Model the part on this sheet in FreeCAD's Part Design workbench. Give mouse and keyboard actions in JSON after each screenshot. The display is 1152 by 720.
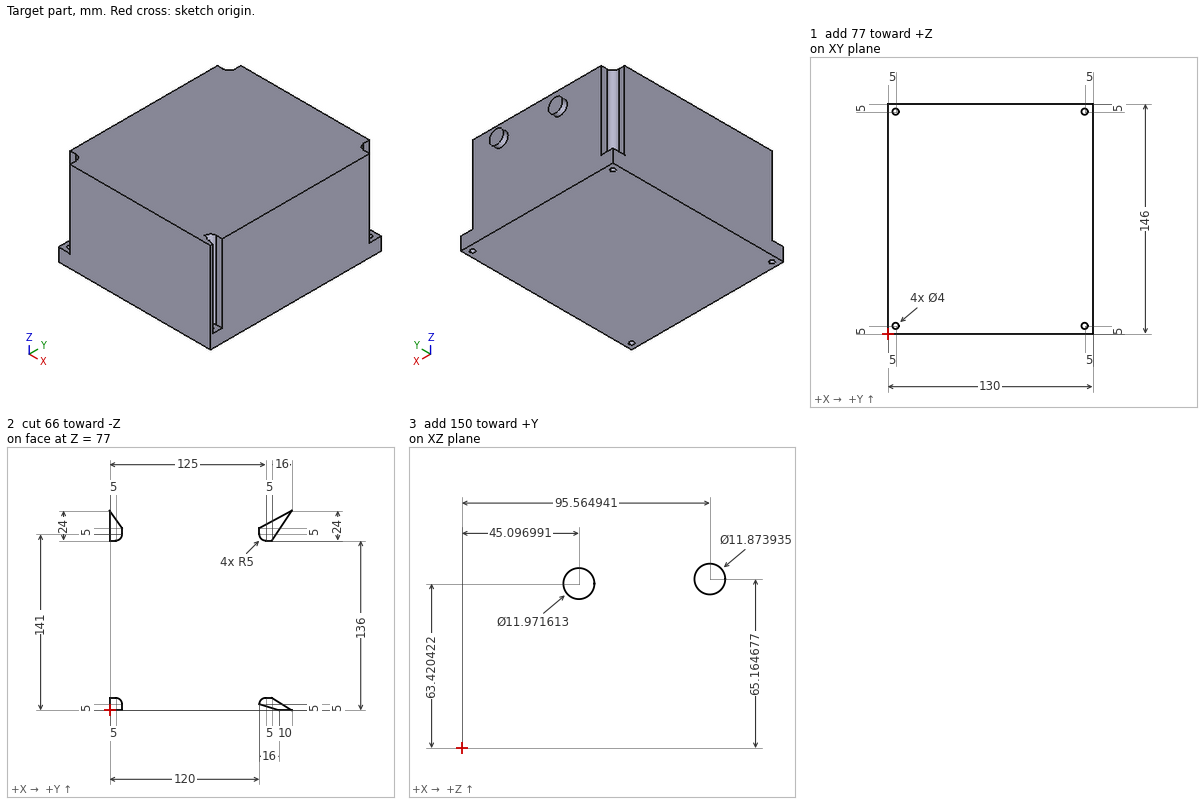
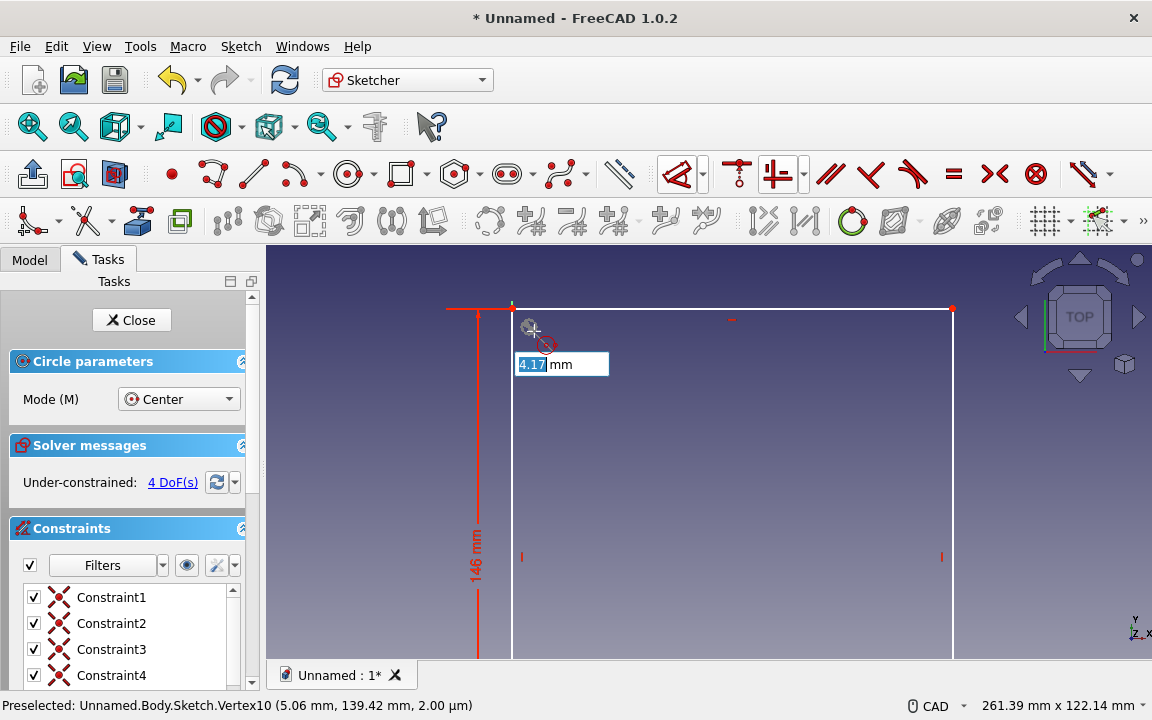
{"action": "type", "text": "4"}
{"action": "key", "text": "Return"}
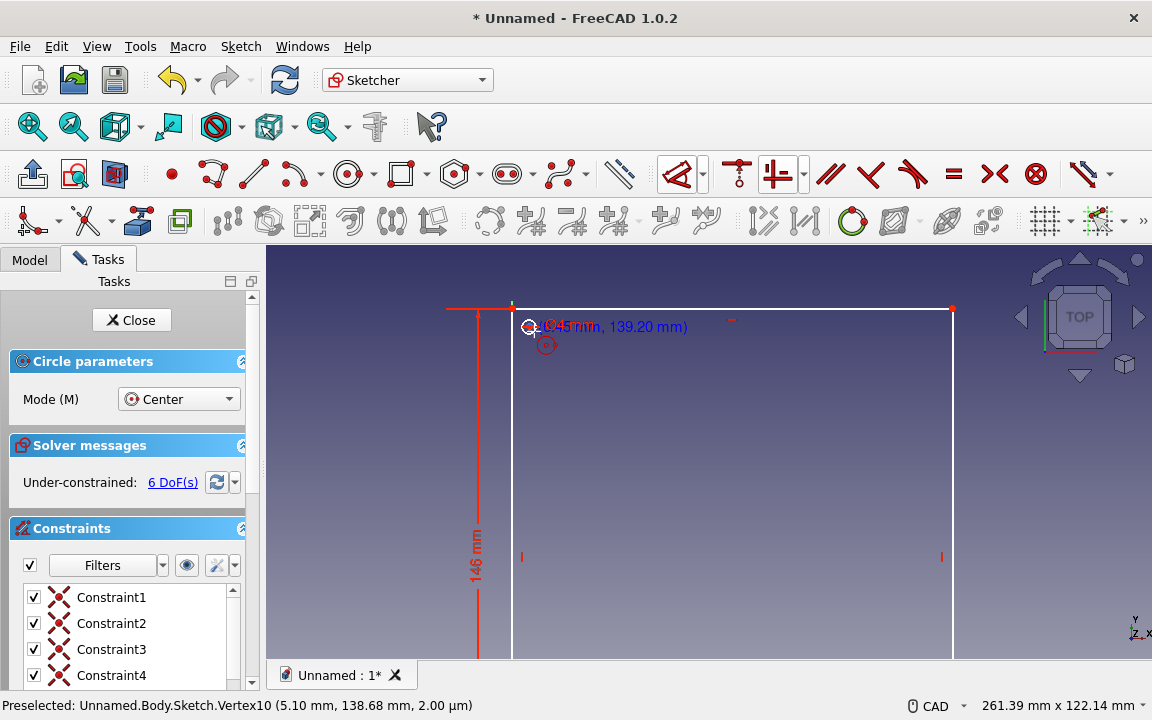
{"action": "scroll", "coordinate": [936, 326], "scroll_direction": "up", "scroll_amount": 7}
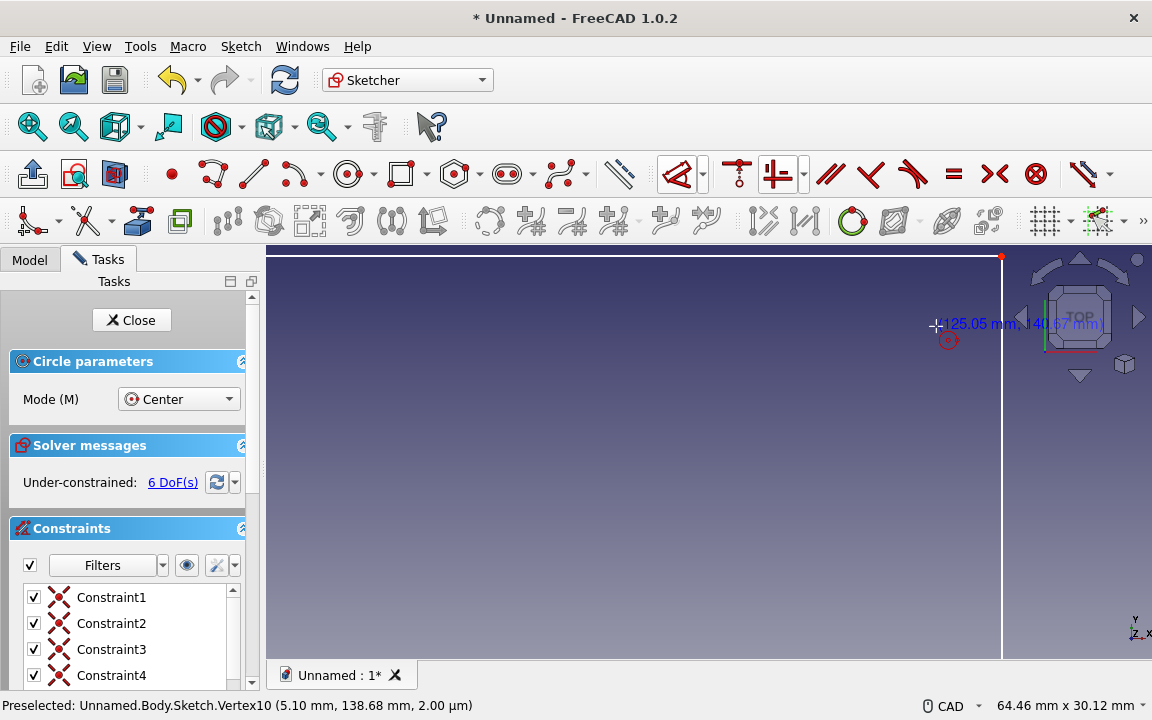
{"action": "scroll", "coordinate": [724, 326], "scroll_direction": "down", "scroll_amount": 10}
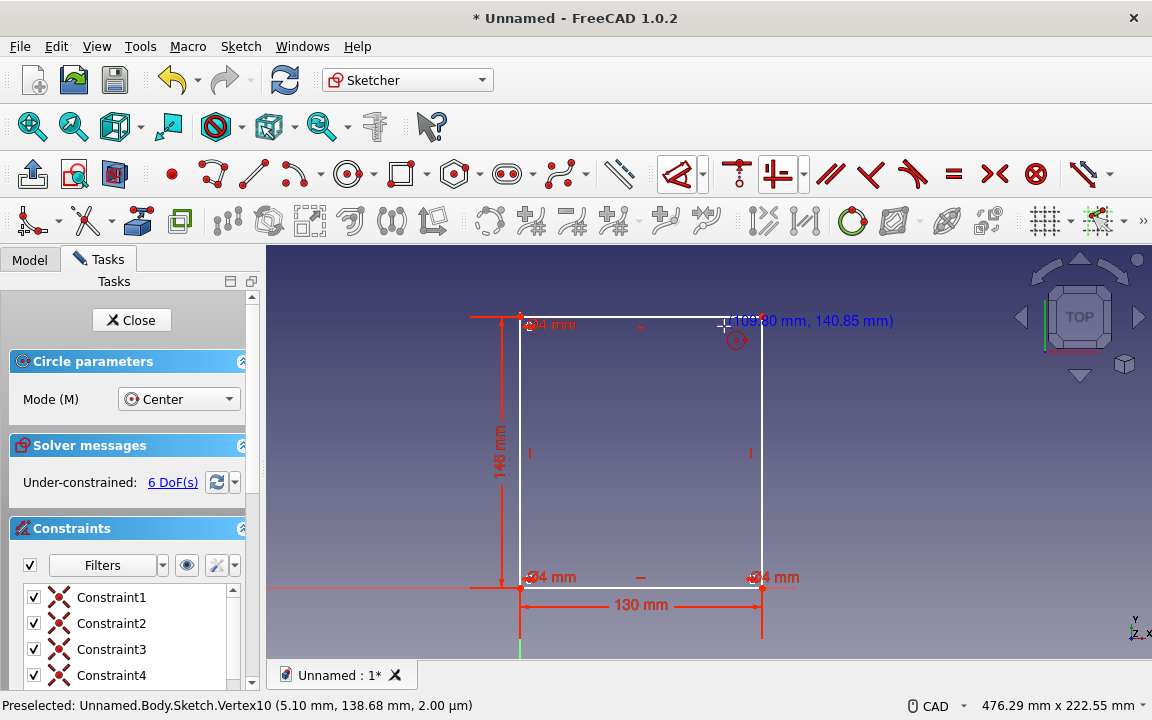
{"action": "scroll", "coordinate": [753, 326], "scroll_direction": "up", "scroll_amount": 3}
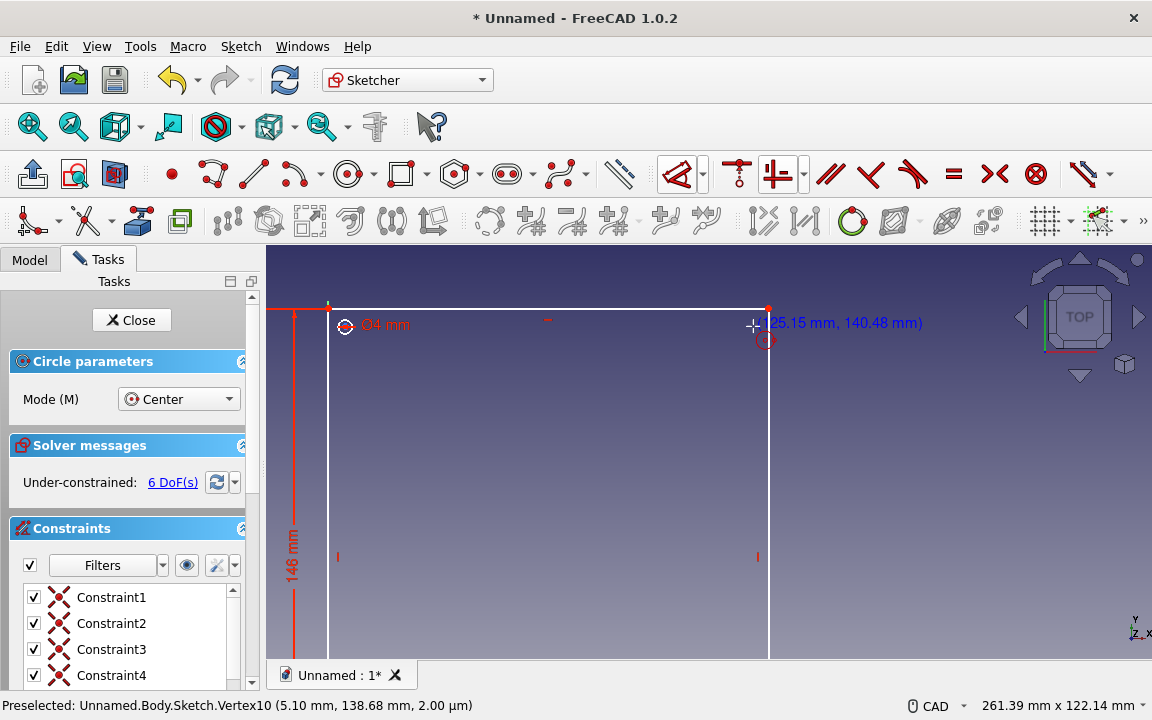
{"action": "left_click", "coordinate": [752, 326]}
{"action": "mouse_move", "coordinate": [747, 331]}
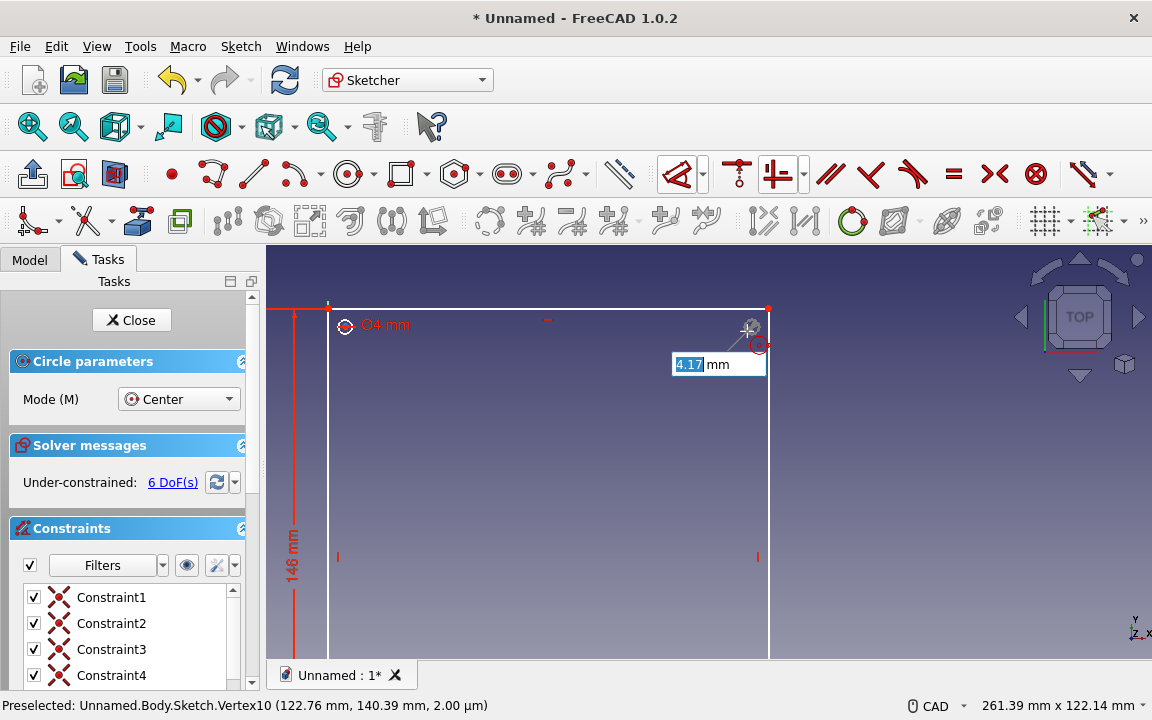
{"action": "type", "text": "4"}
{"action": "key", "text": "Return"}
{"action": "key", "text": "Escape"}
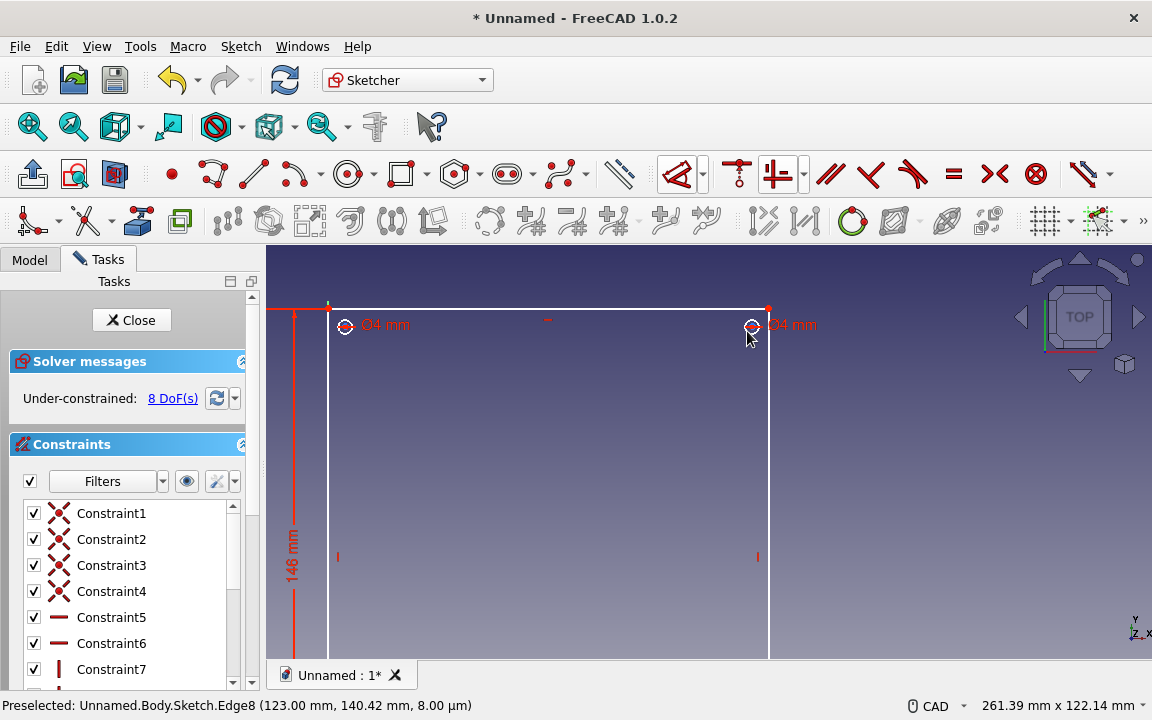
{"action": "left_click", "coordinate": [676, 174]}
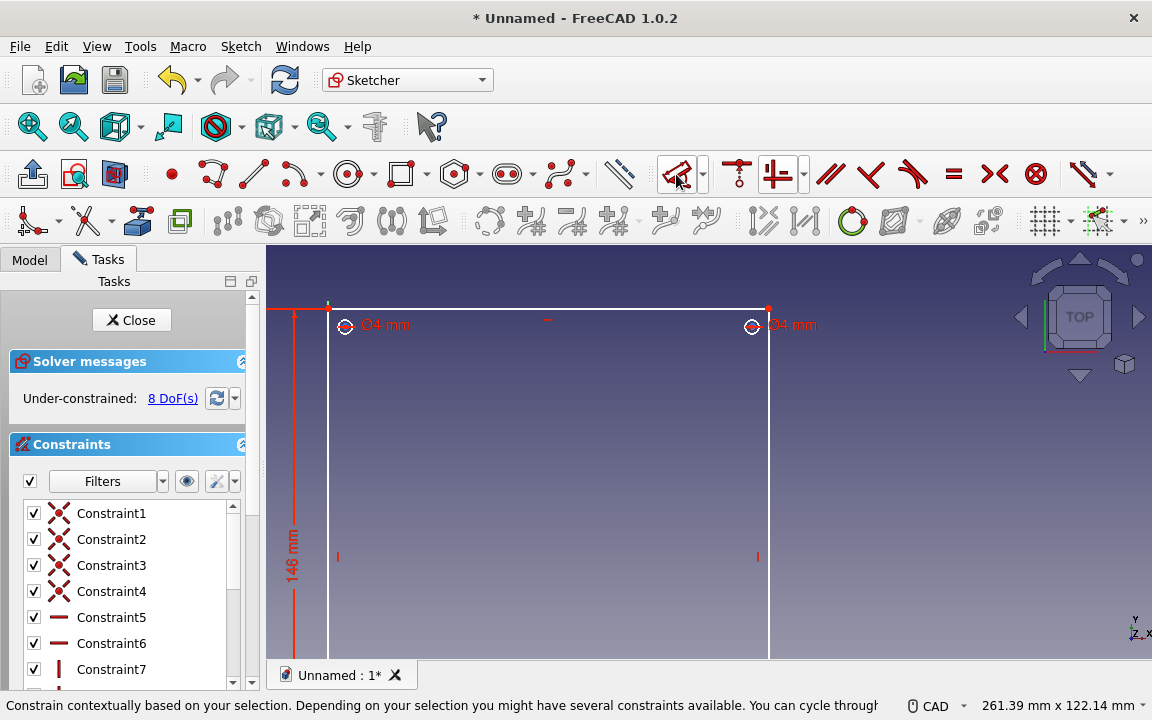
{"action": "scroll", "coordinate": [752, 325], "scroll_direction": "down", "scroll_amount": 3}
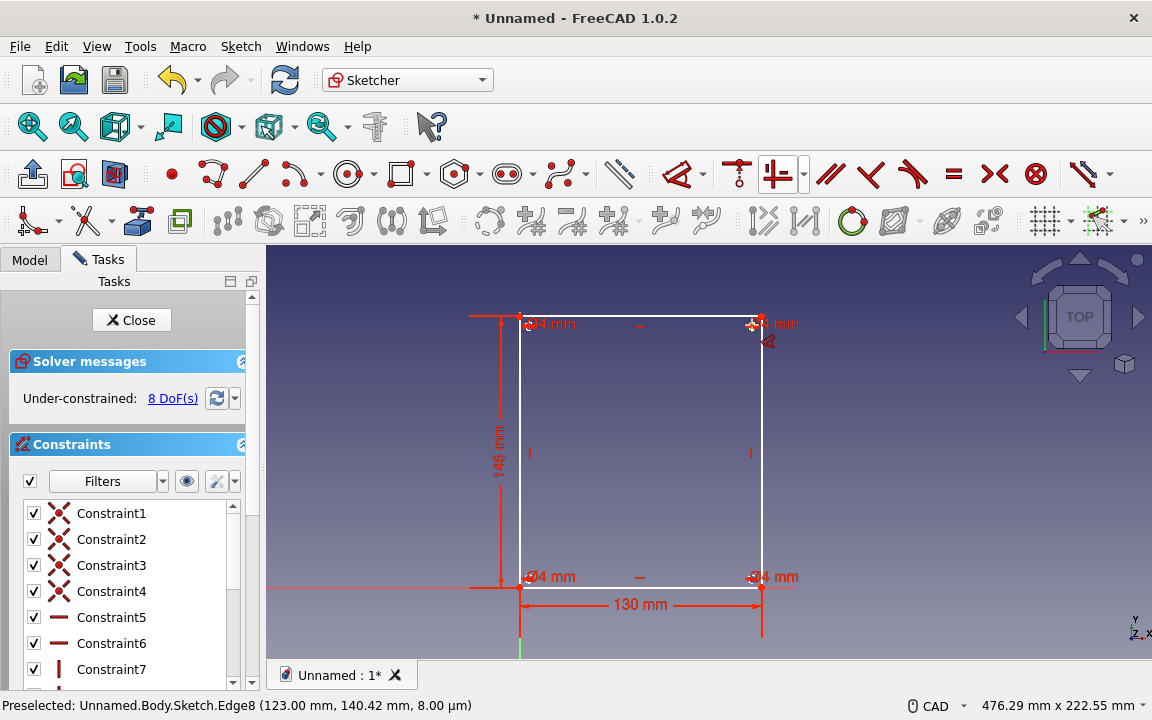
{"action": "scroll", "coordinate": [529, 579], "scroll_direction": "up", "scroll_amount": 8}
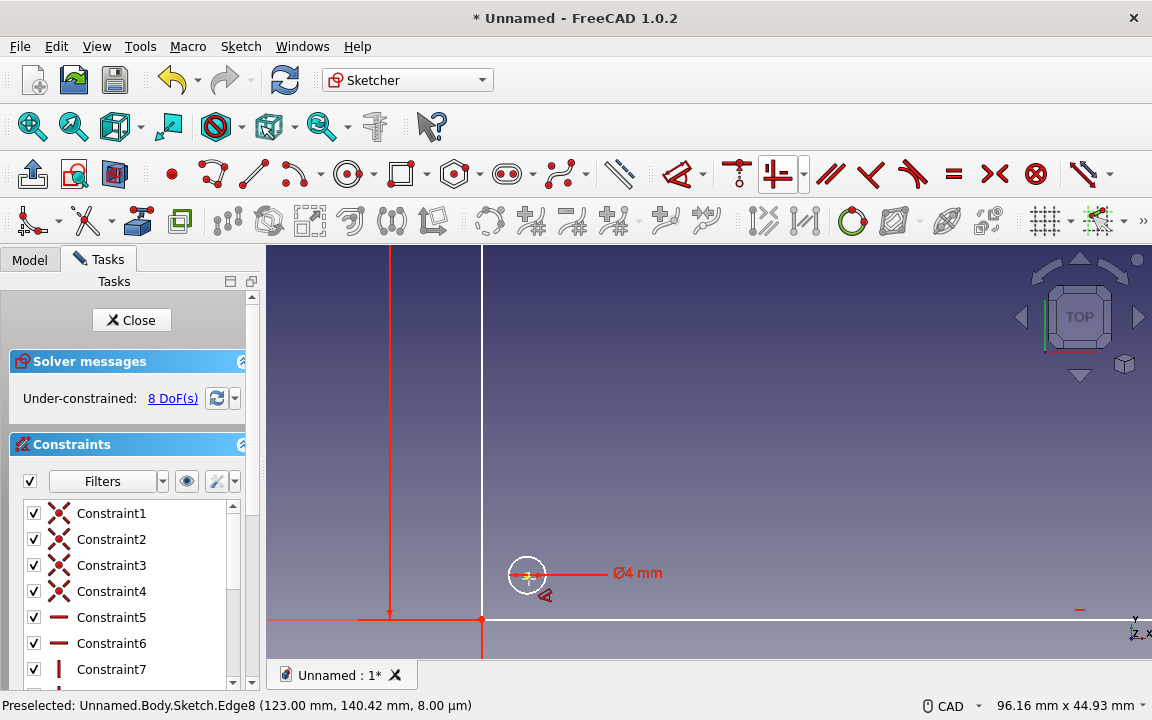
{"action": "left_click", "coordinate": [527, 575]}
{"action": "left_click", "coordinate": [505, 541]}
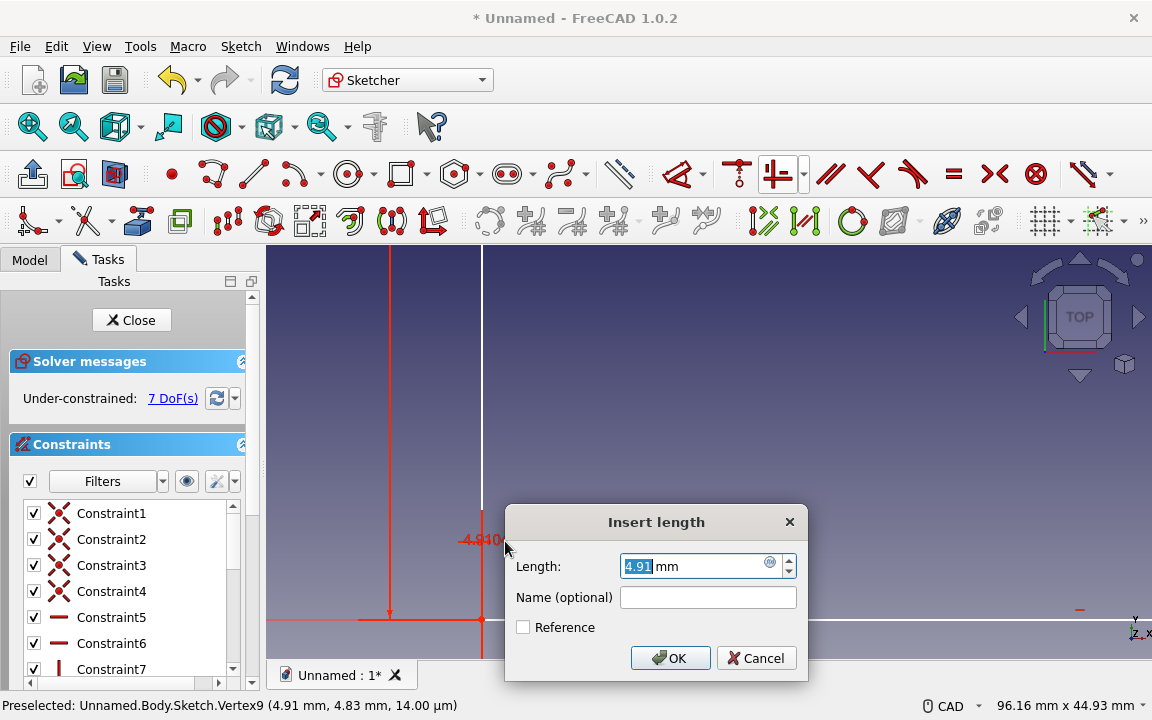
{"action": "type", "text": "5"}
{"action": "key", "text": "Return"}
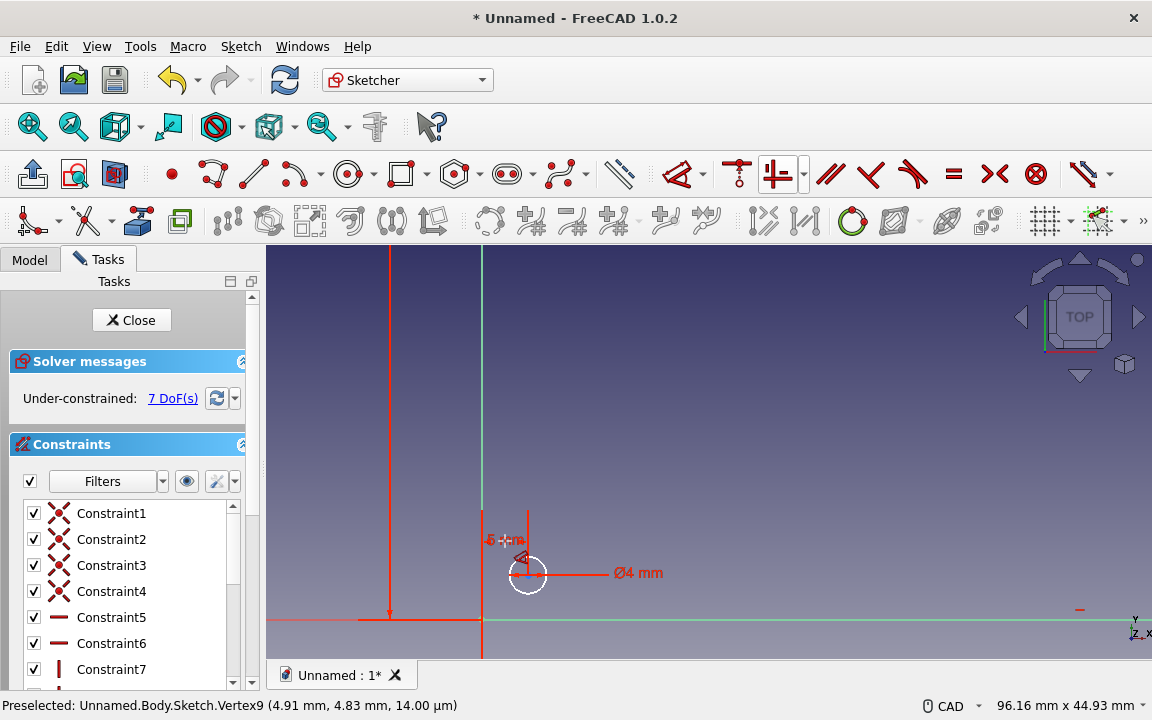
{"action": "left_click", "coordinate": [528, 575]}
{"action": "left_click", "coordinate": [448, 597]}